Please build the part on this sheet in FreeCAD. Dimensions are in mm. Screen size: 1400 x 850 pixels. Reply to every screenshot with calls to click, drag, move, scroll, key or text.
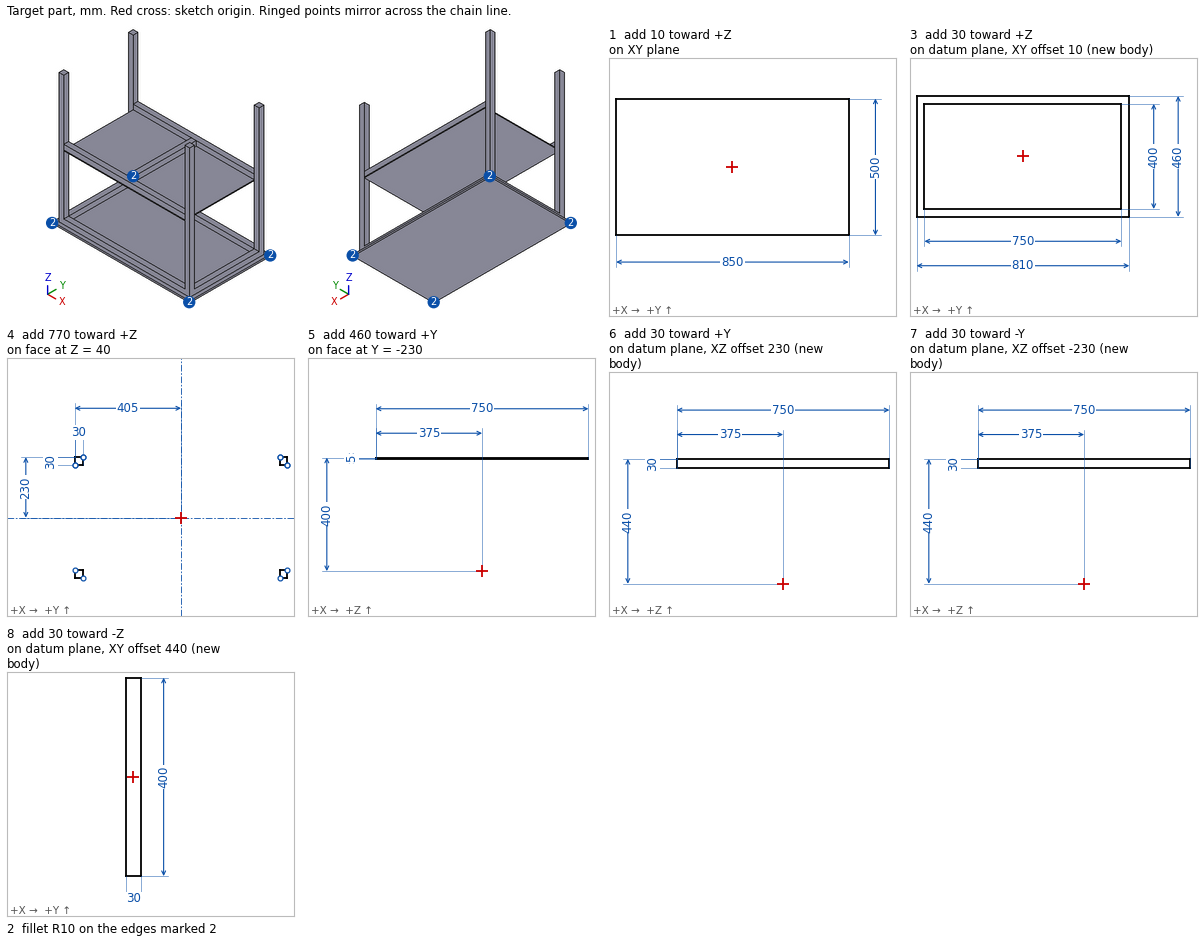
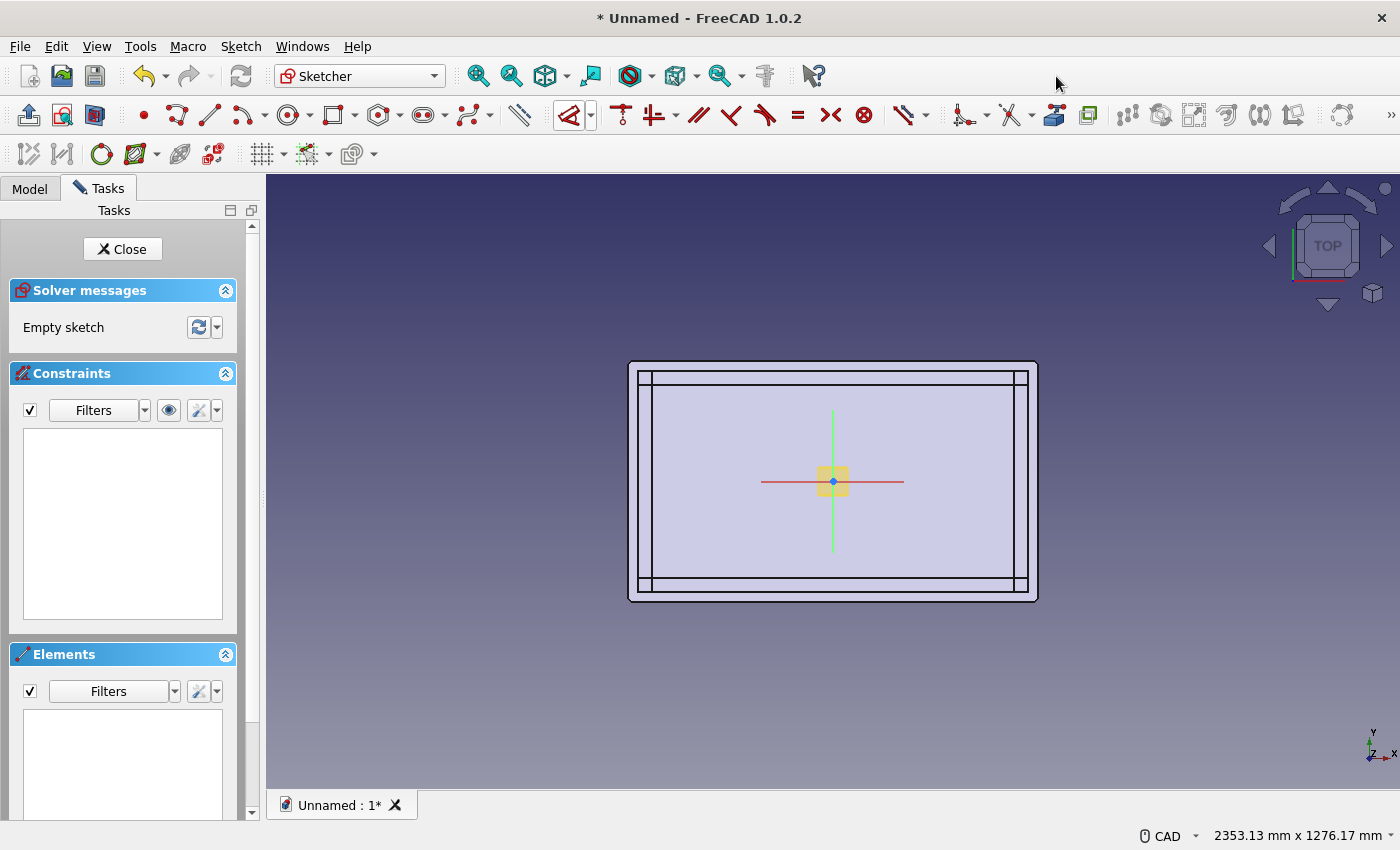
scroll(889, 482, up, 4)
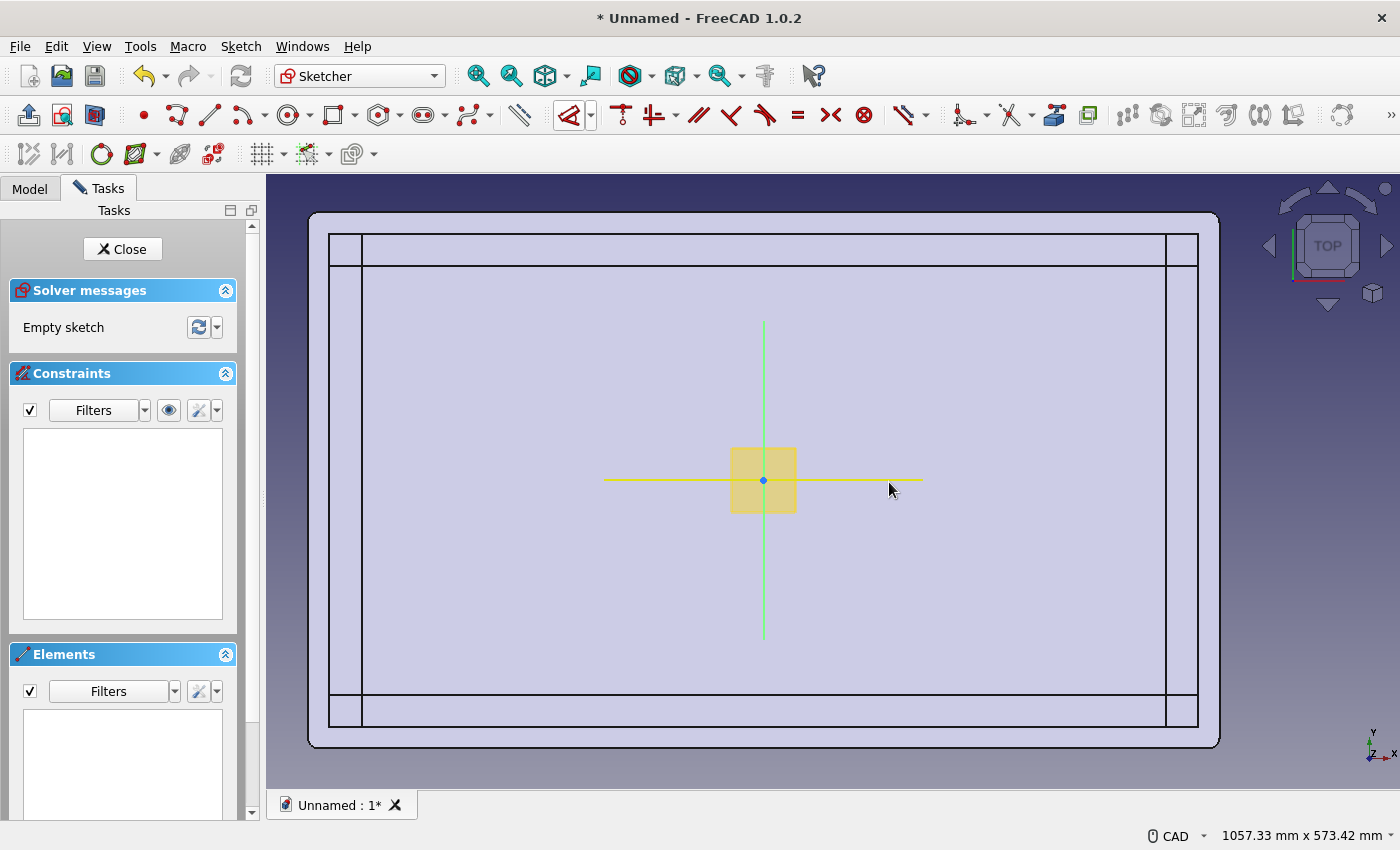
click(354, 116)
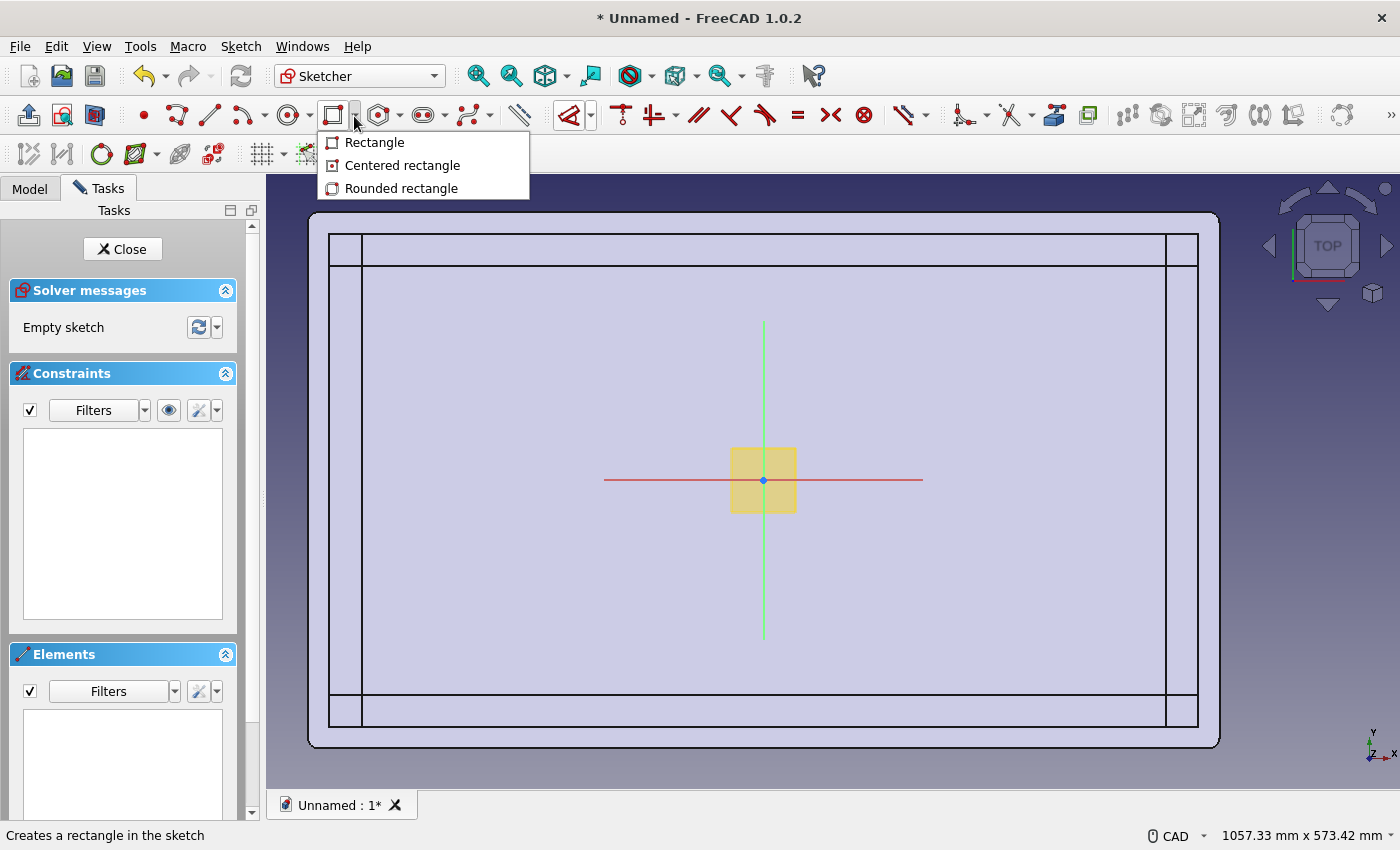
click(424, 166)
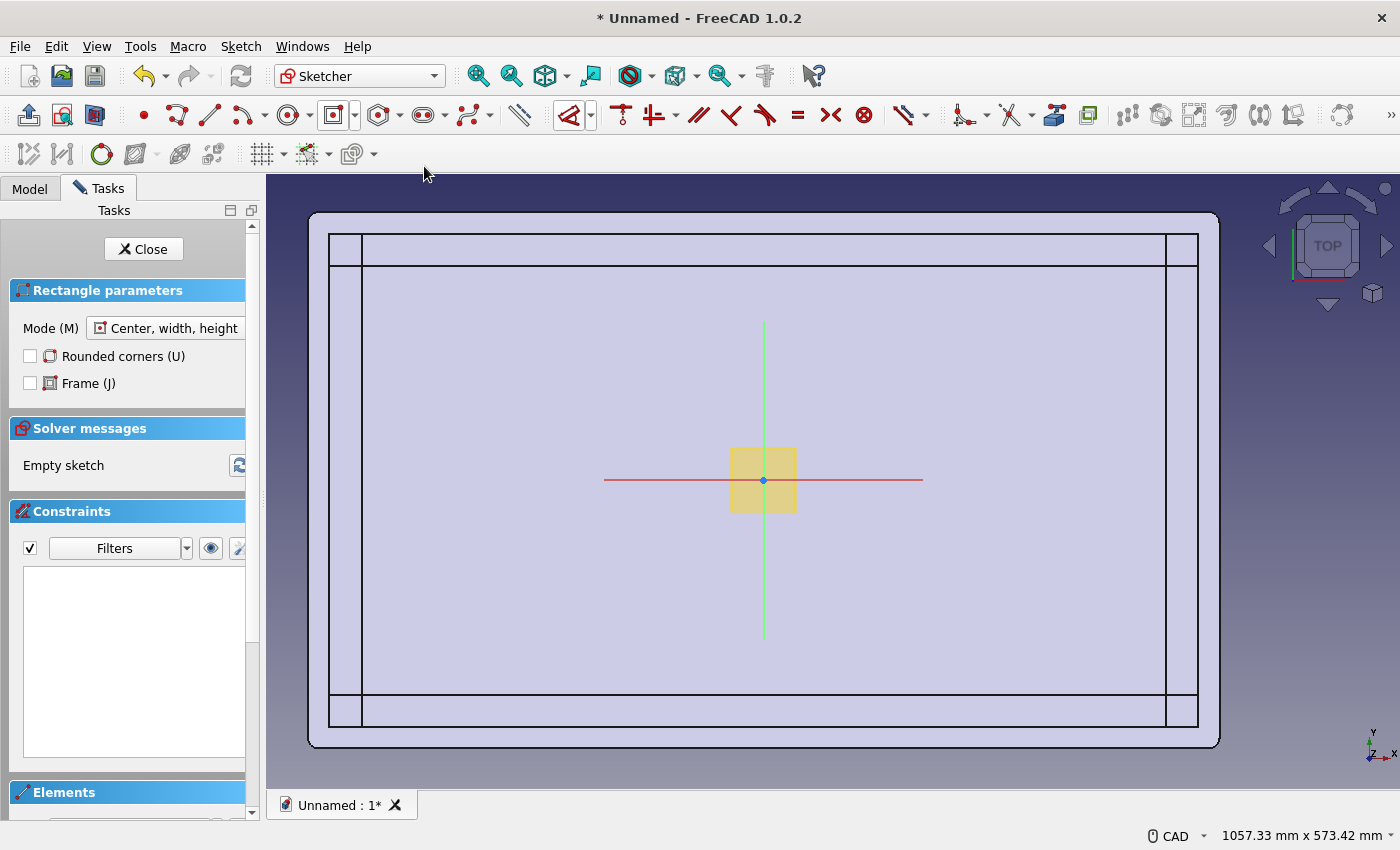
click(764, 480)
click(780, 266)
key(Escape)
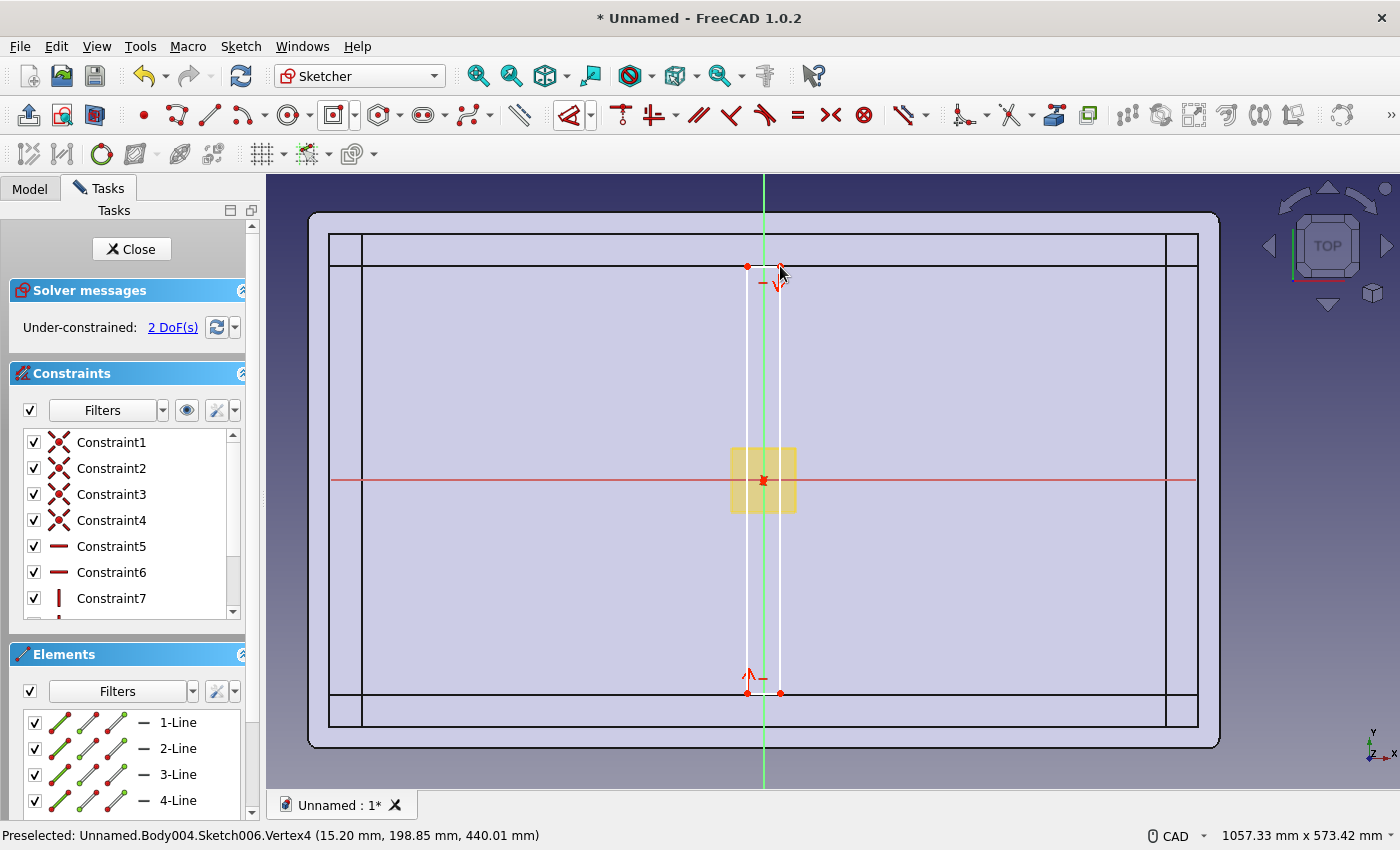
scroll(760, 694, up, 2)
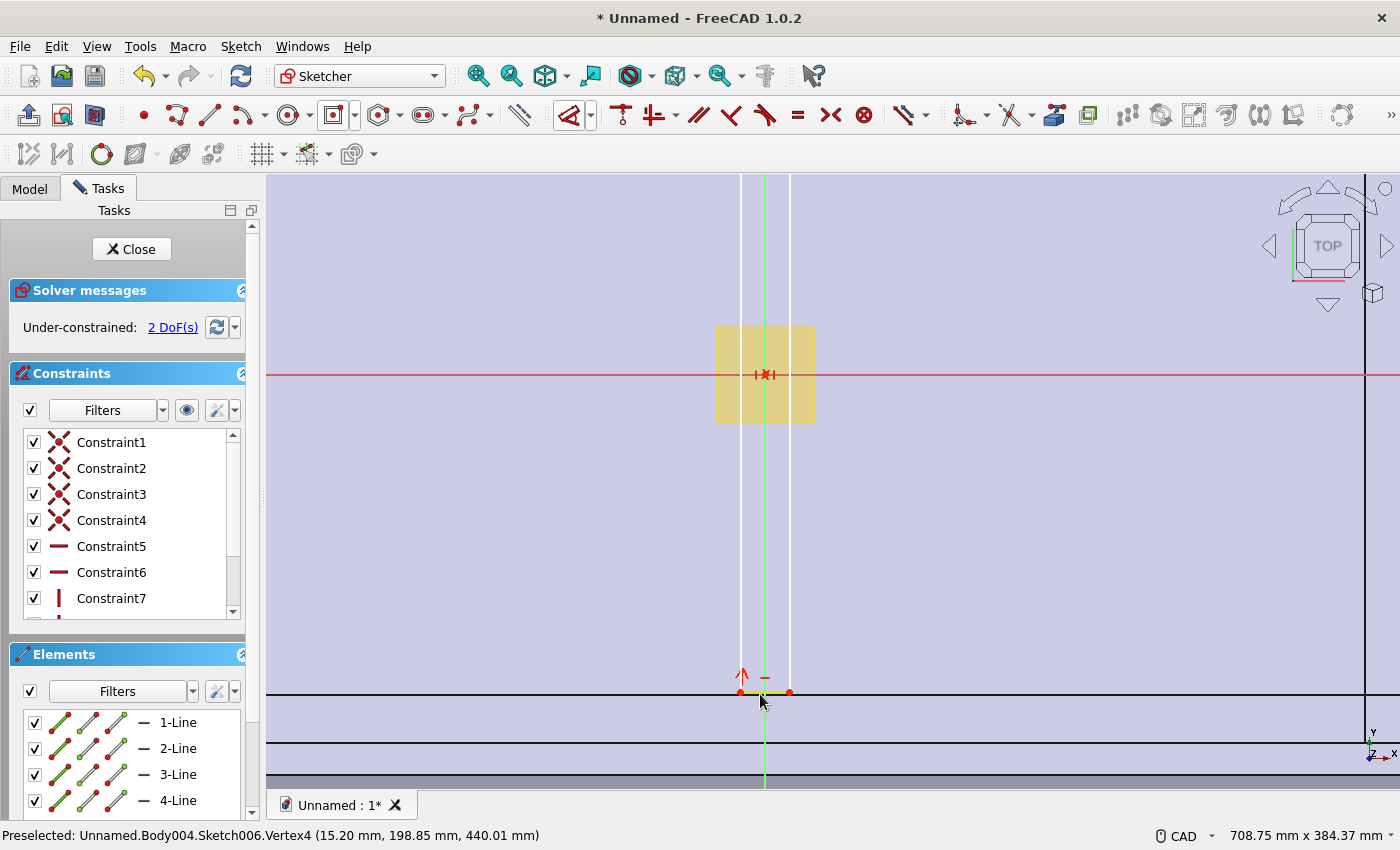
click(760, 693)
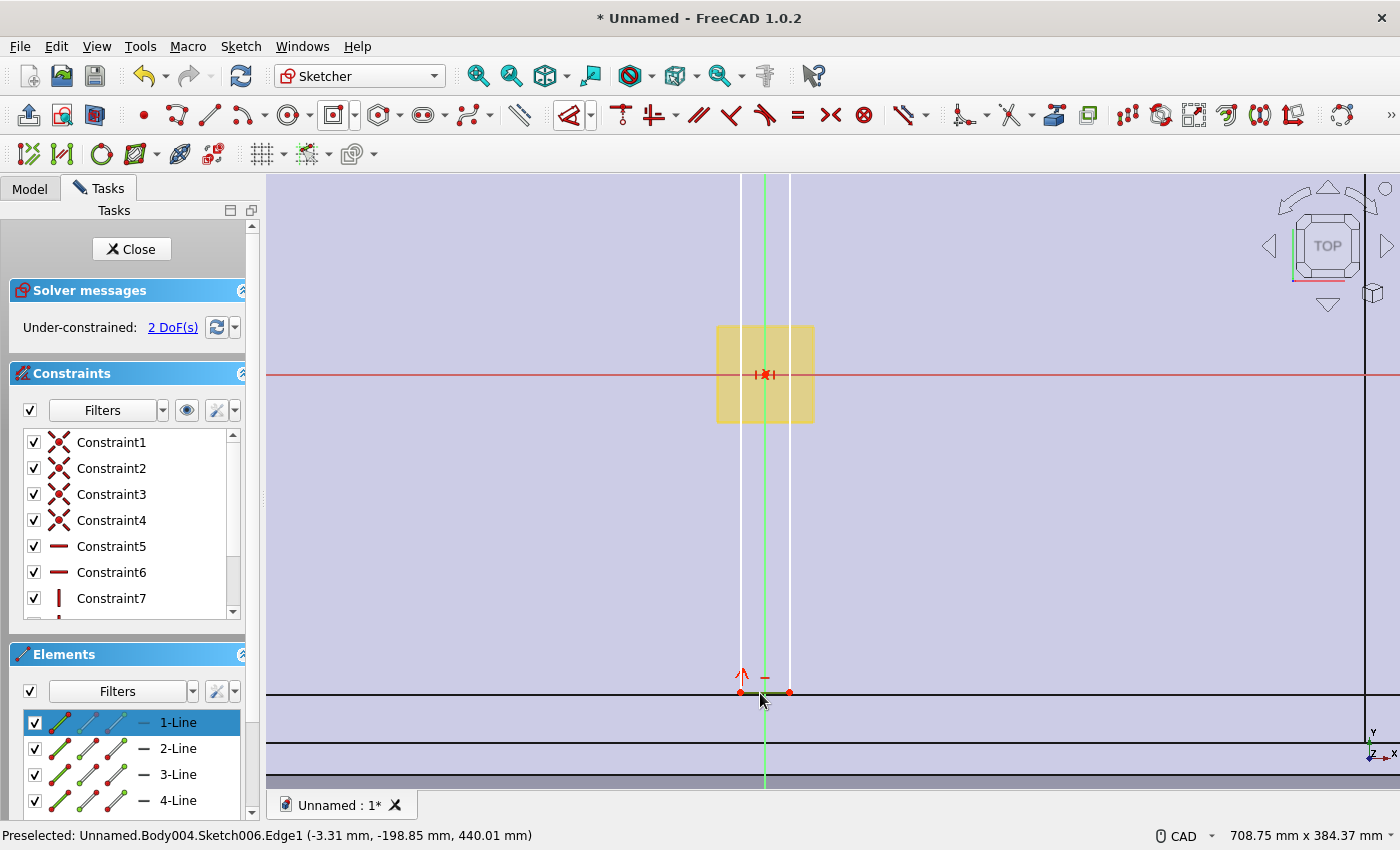
key(l)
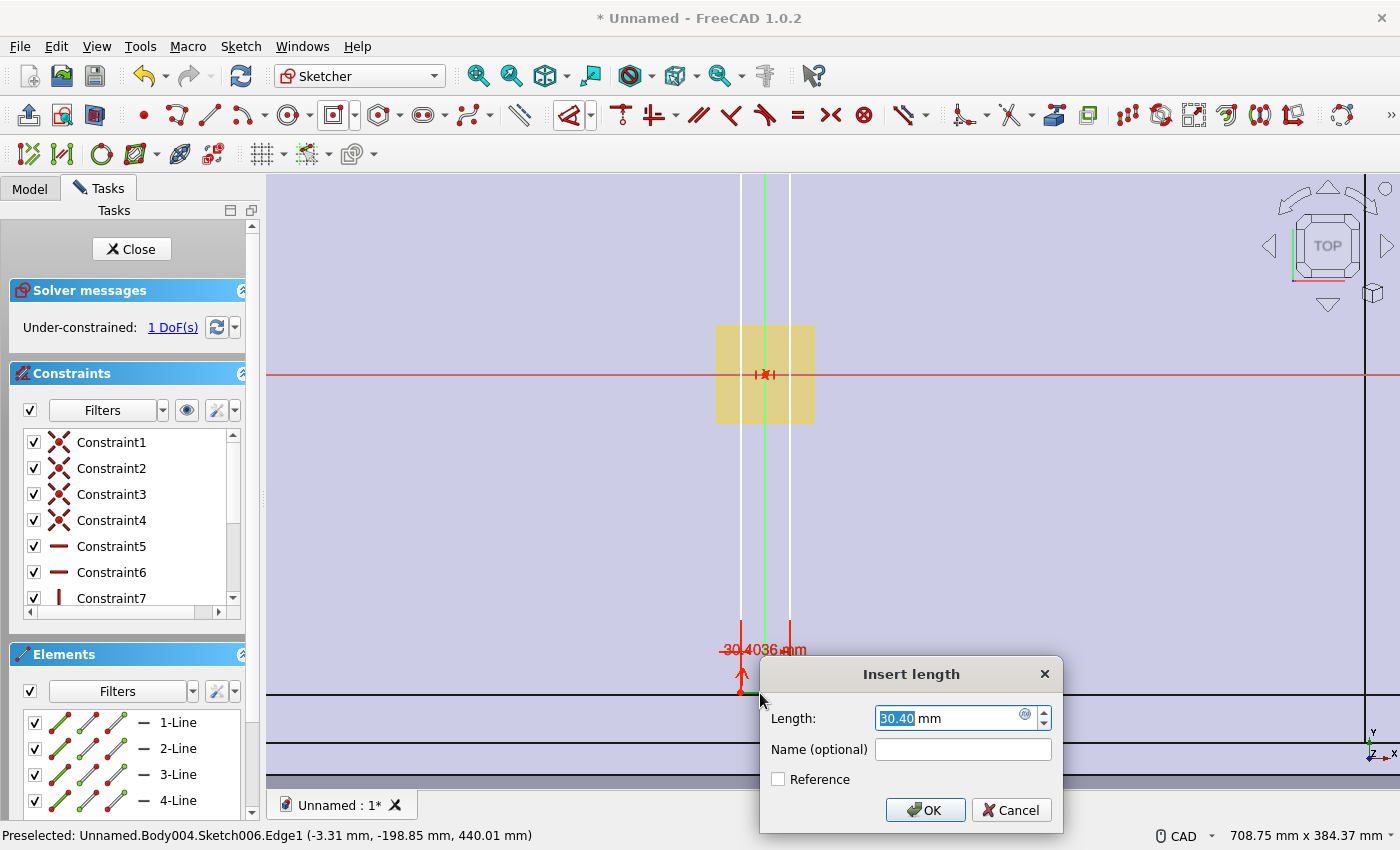
text(30)
key(Return)